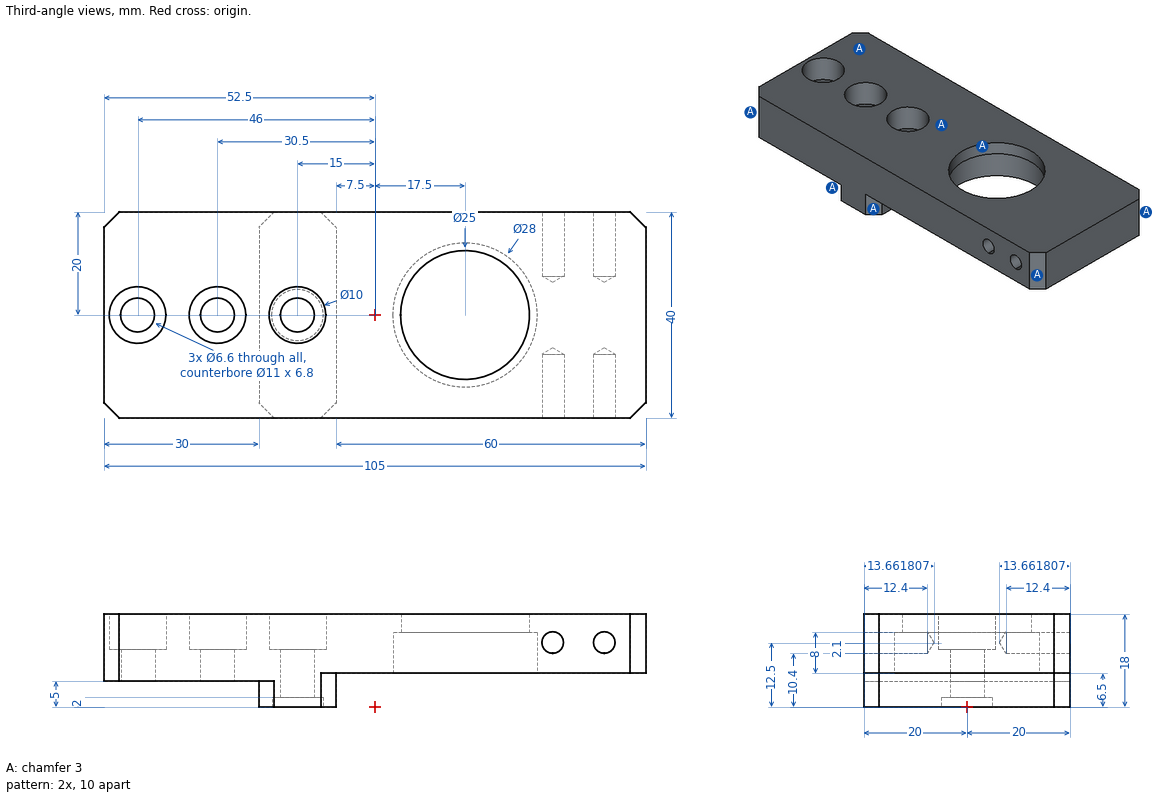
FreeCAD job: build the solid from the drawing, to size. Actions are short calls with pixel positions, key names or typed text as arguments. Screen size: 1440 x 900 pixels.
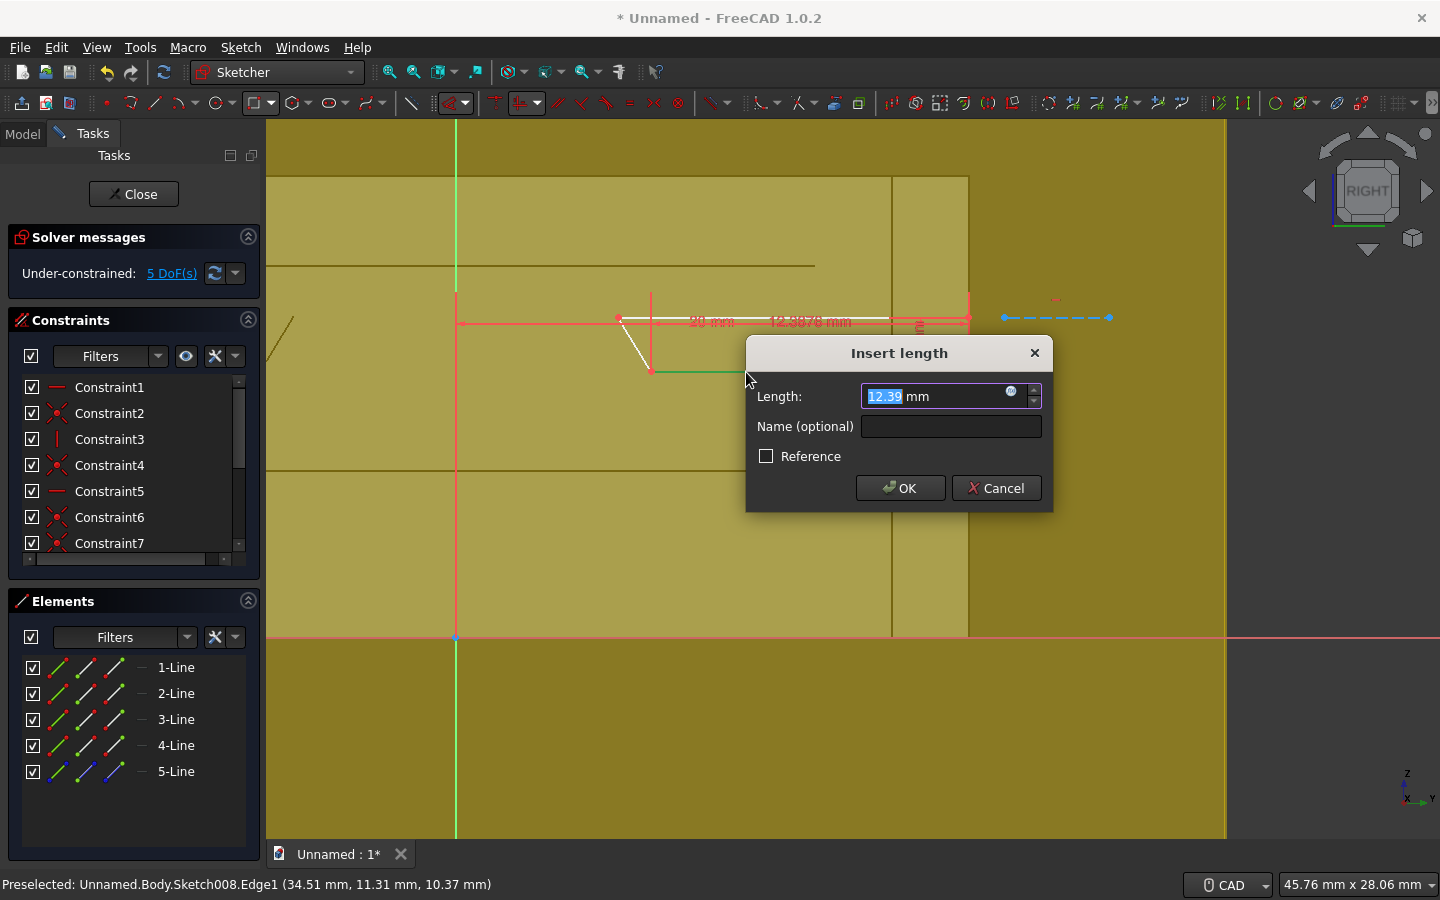
text(12.4)
key(Return)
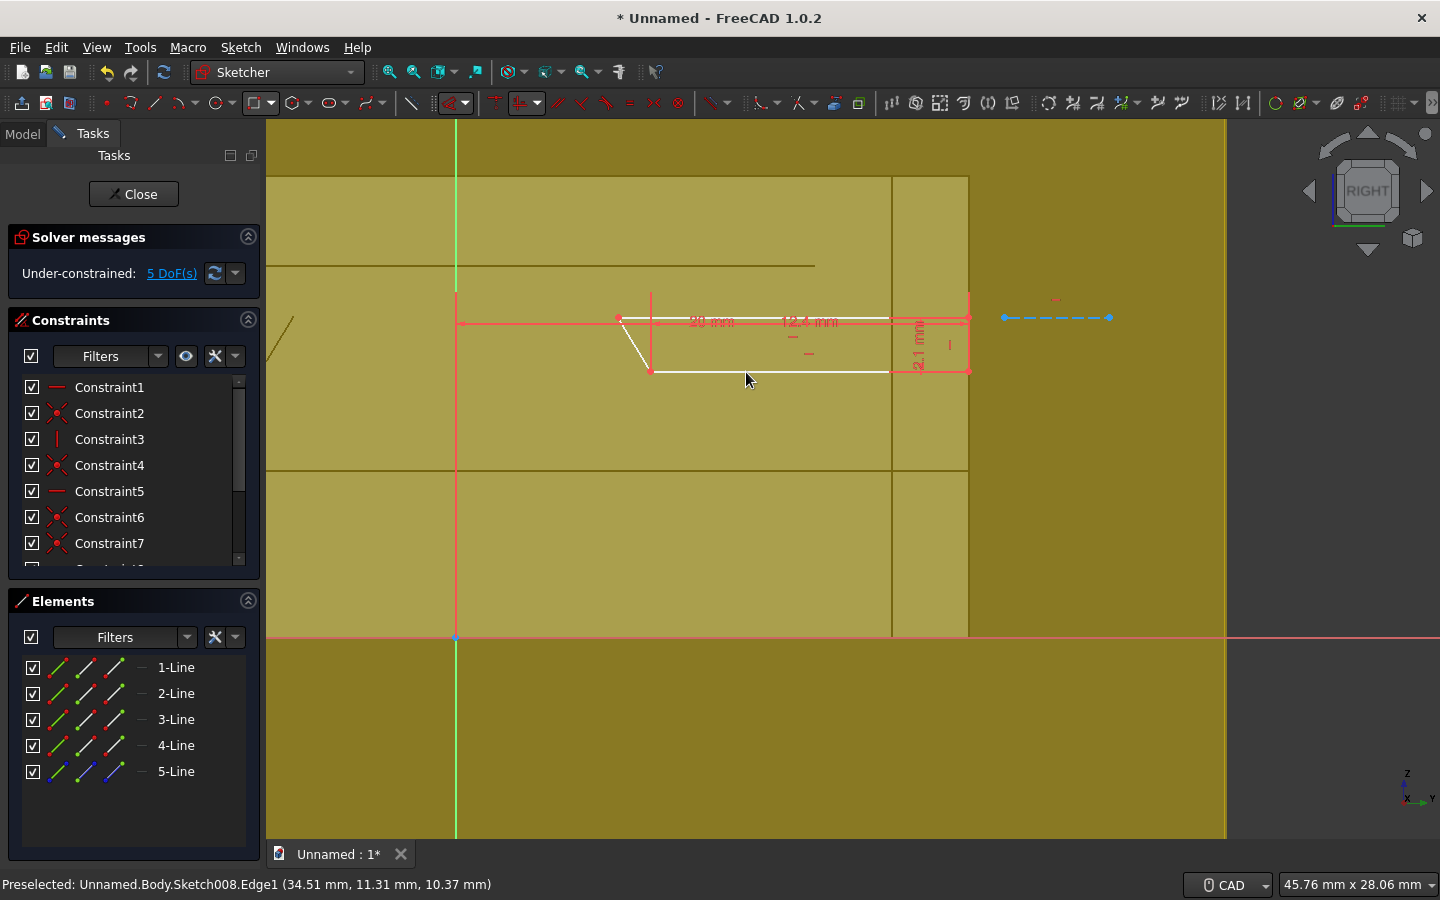
click(651, 372)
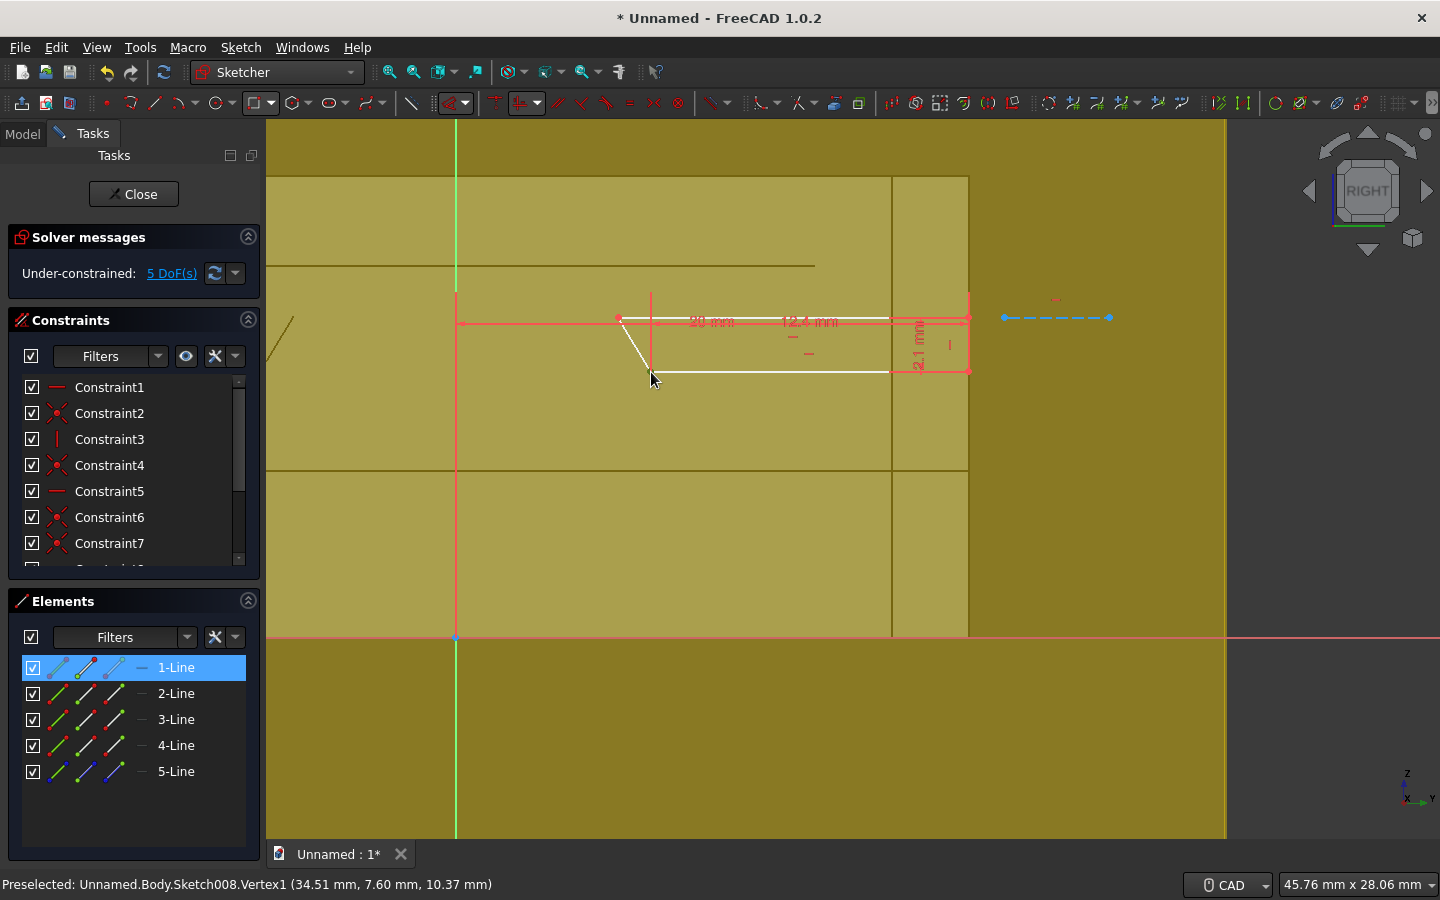
click(468, 104)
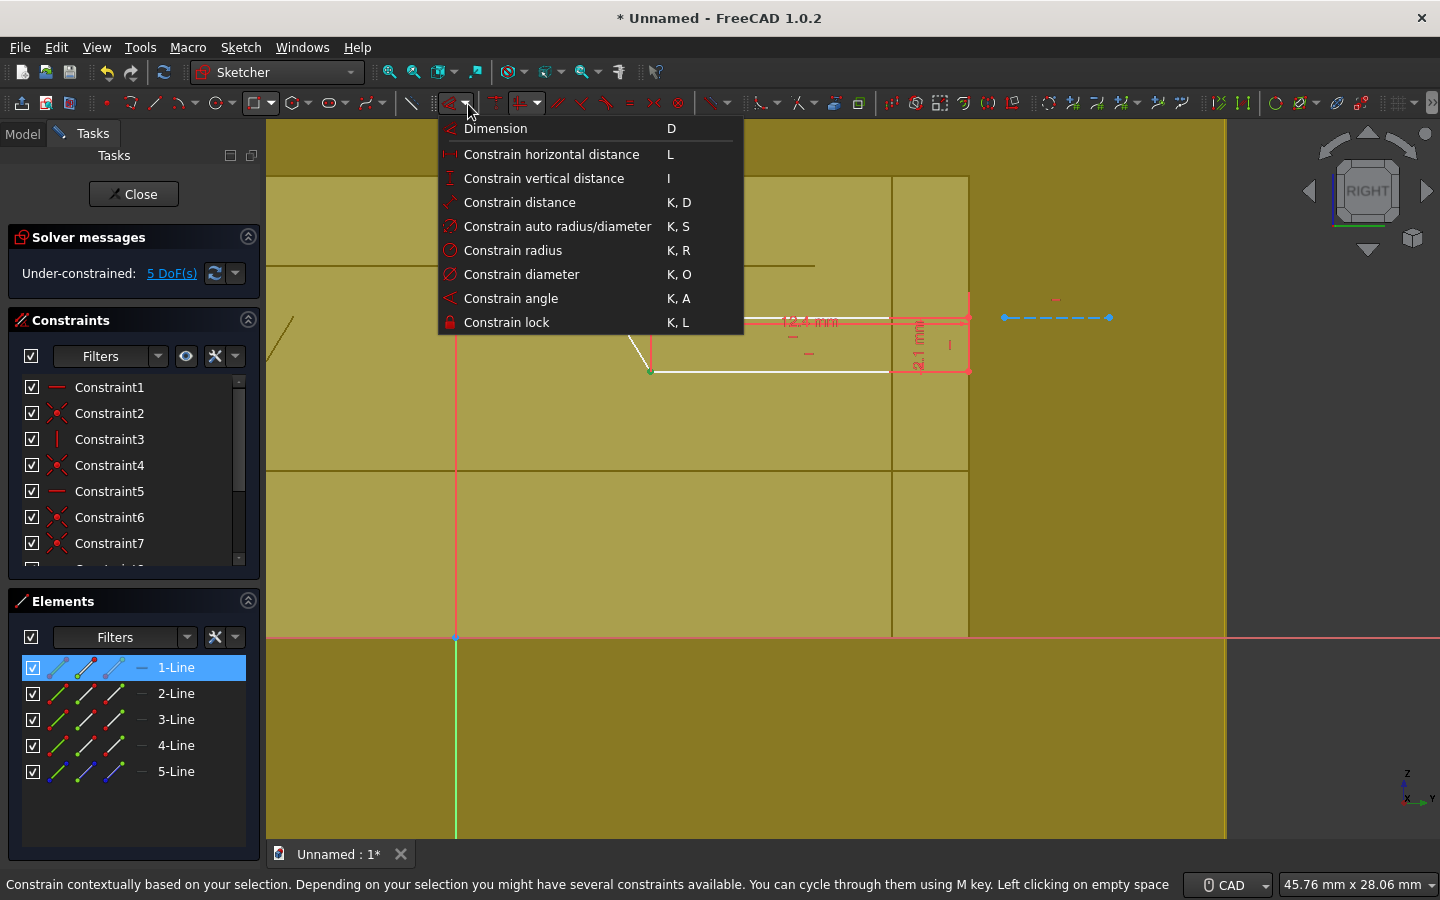
click(591, 178)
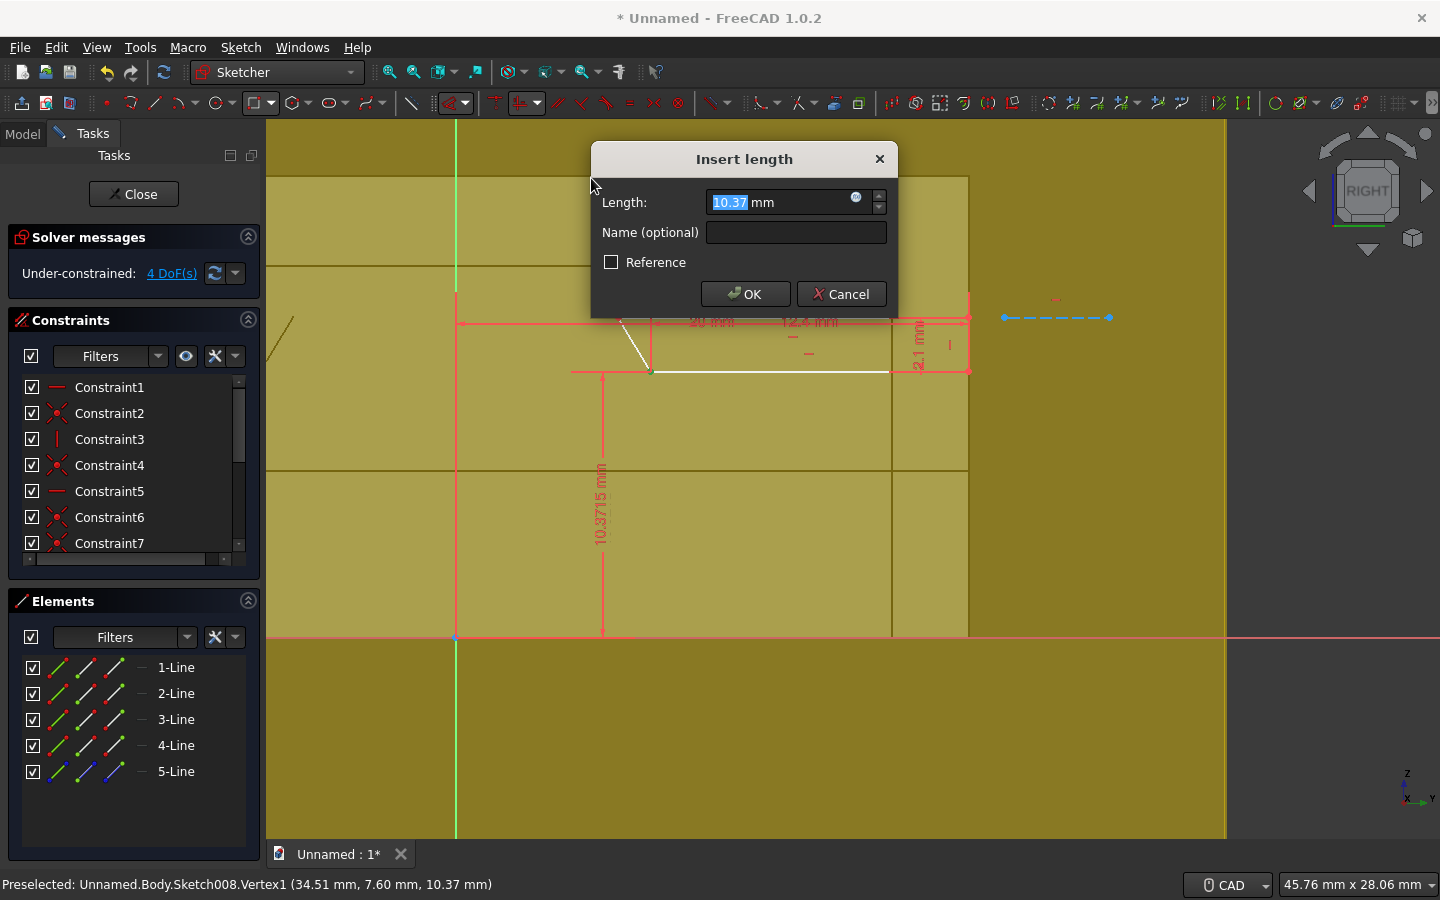
text(10.4)
key(Return)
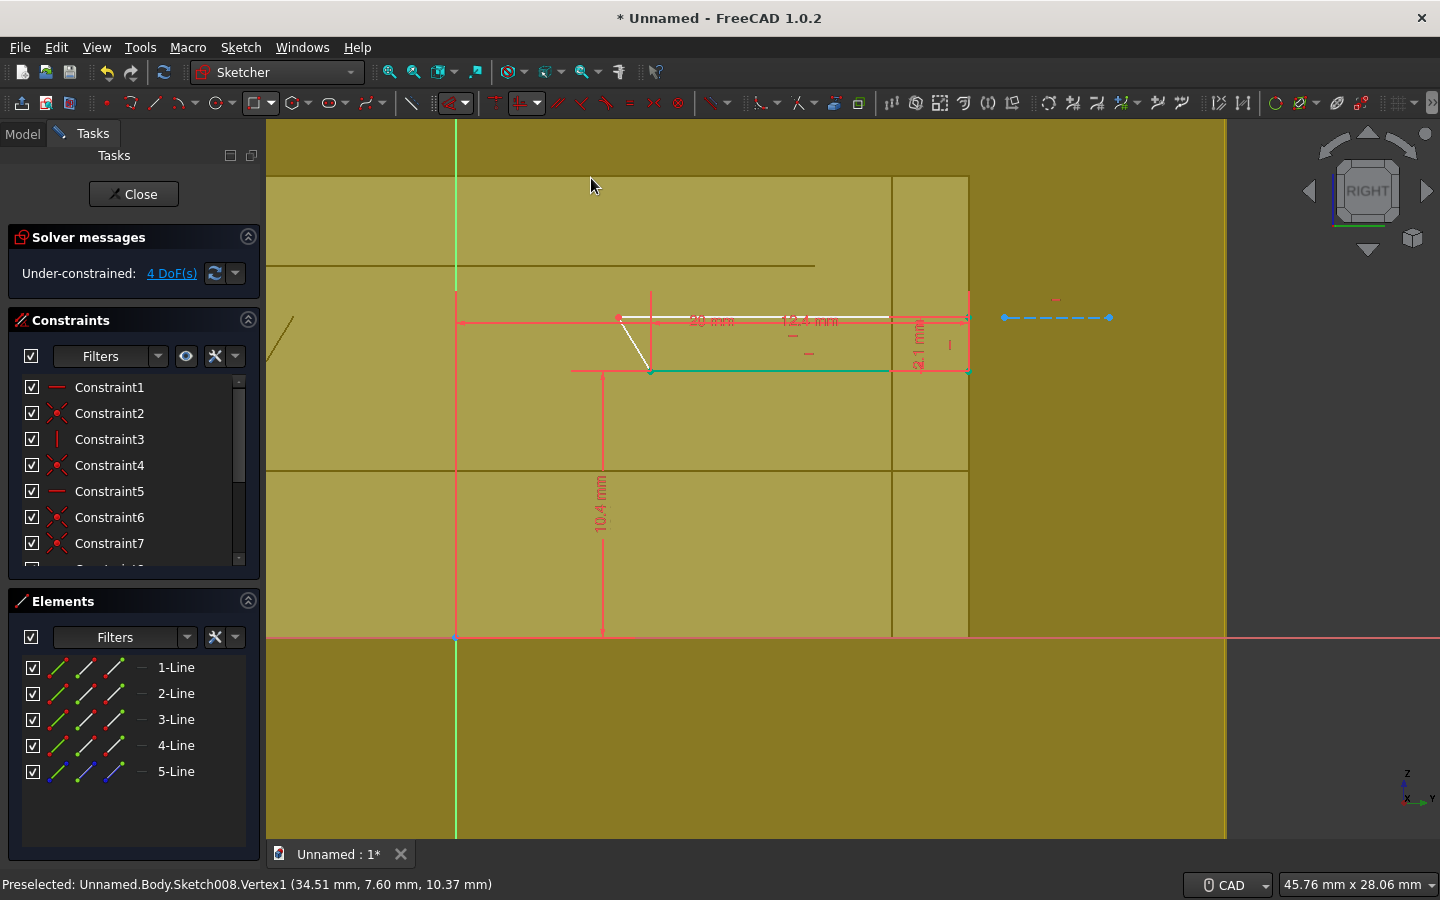
click(1004, 318)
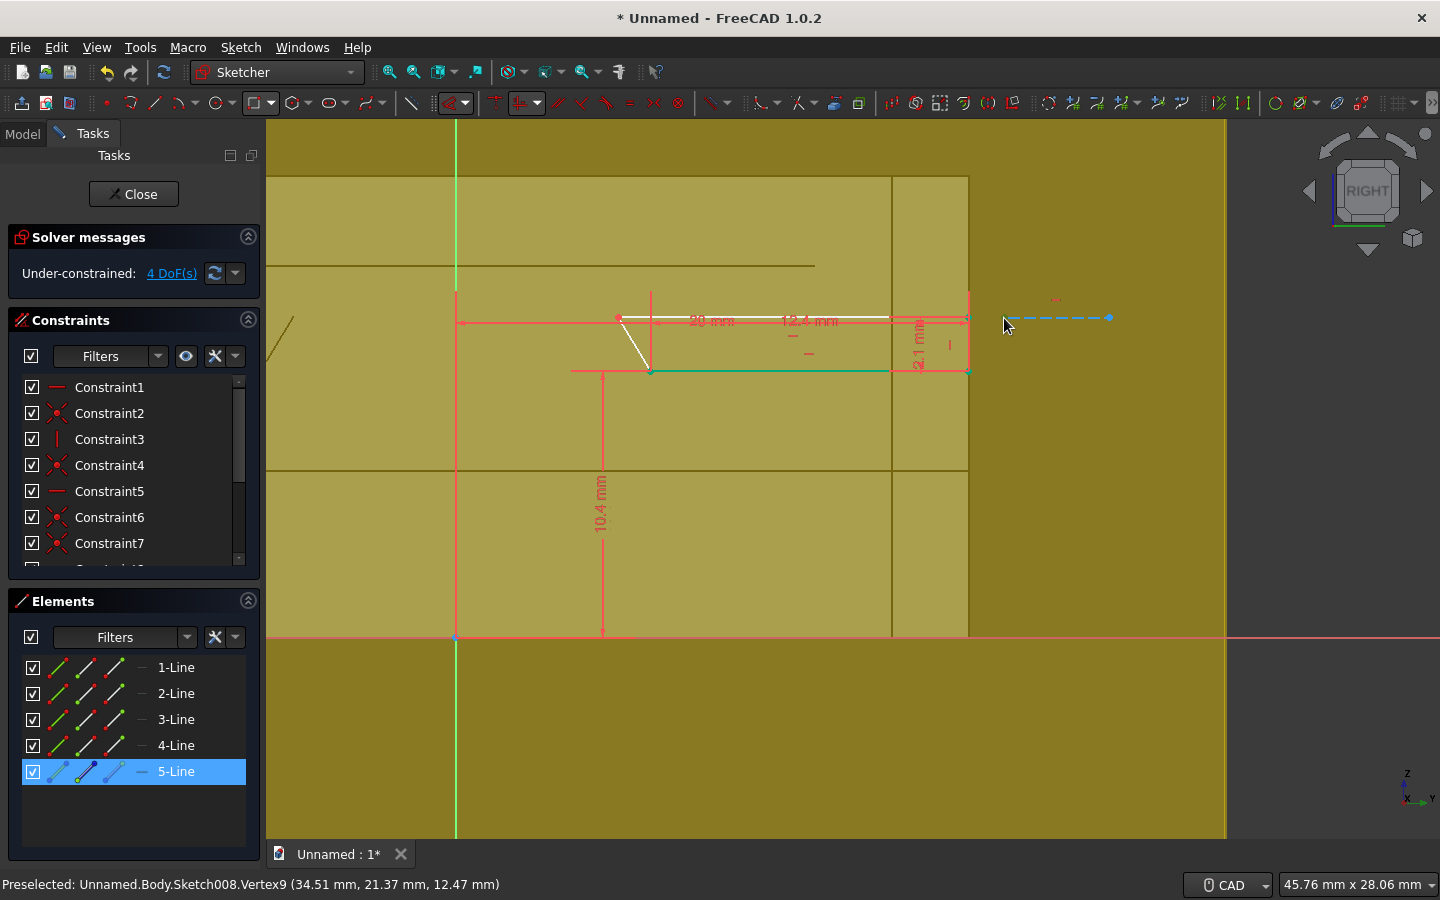
click(468, 104)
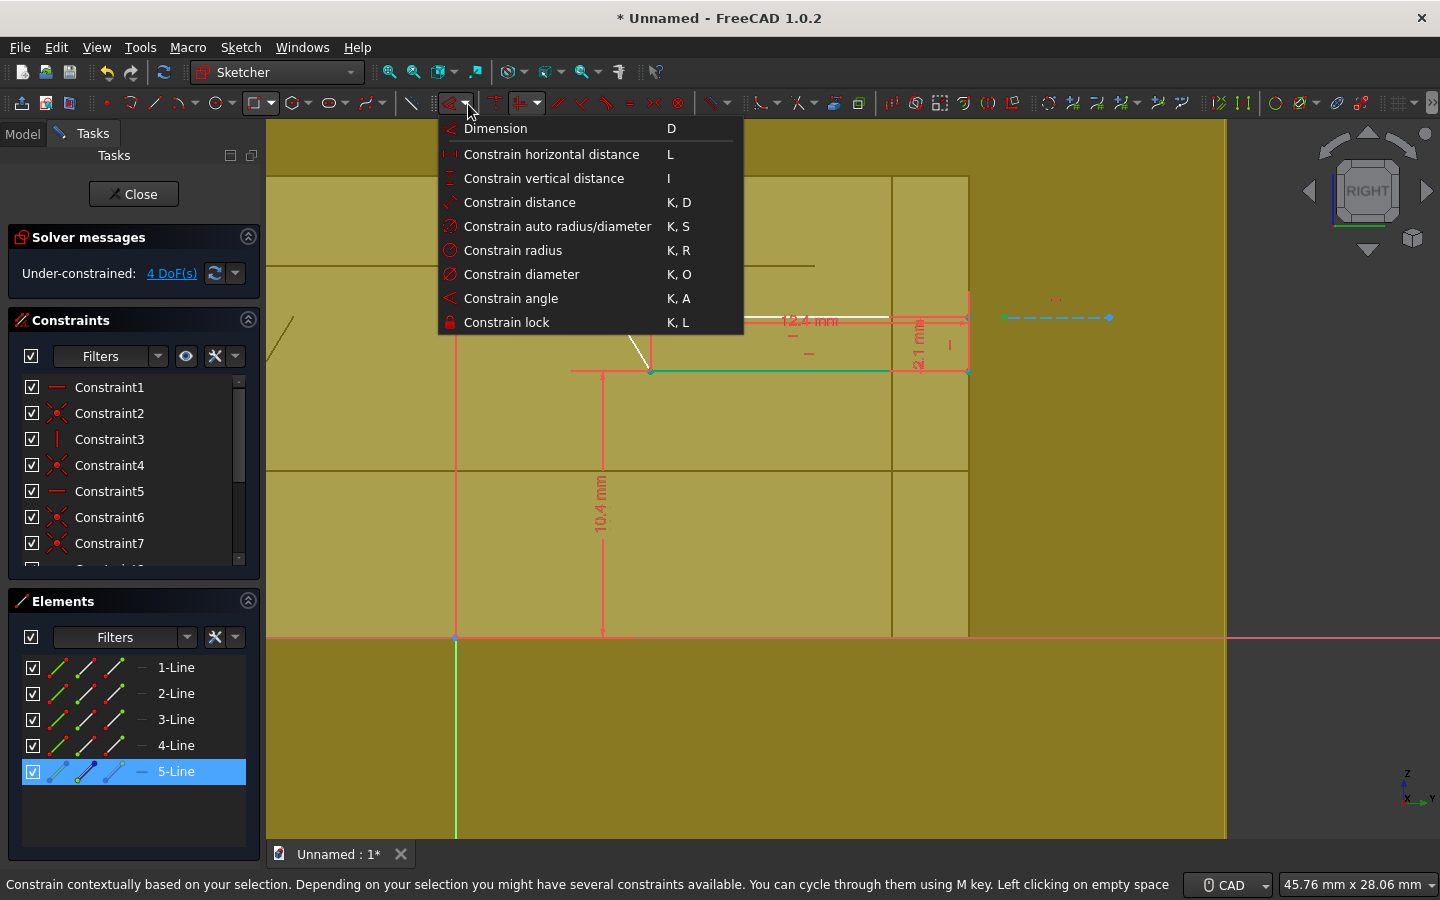
click(591, 178)